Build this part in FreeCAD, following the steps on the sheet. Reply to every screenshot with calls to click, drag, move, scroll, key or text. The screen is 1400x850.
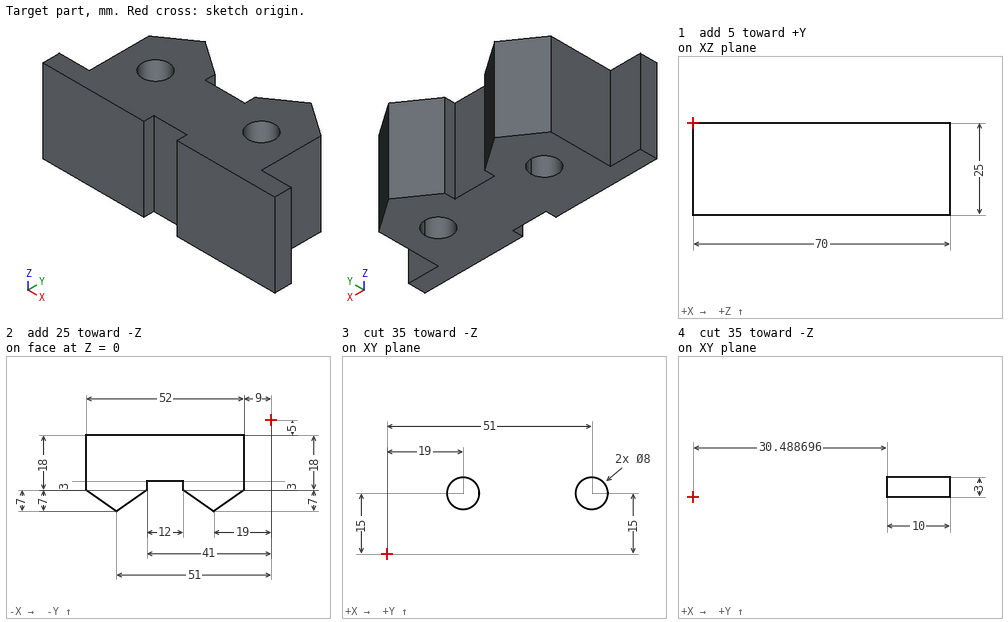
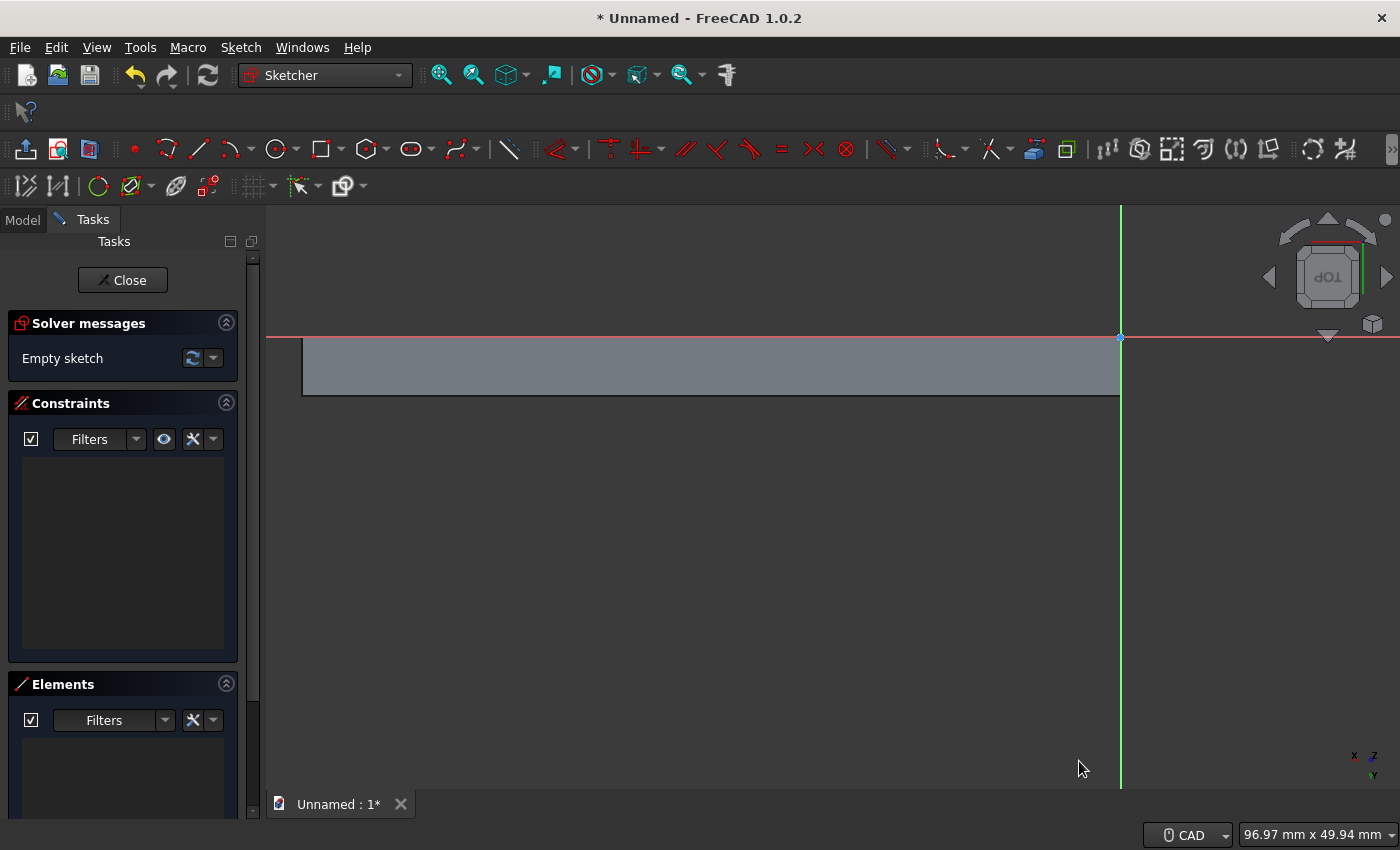
key(g)
key(m)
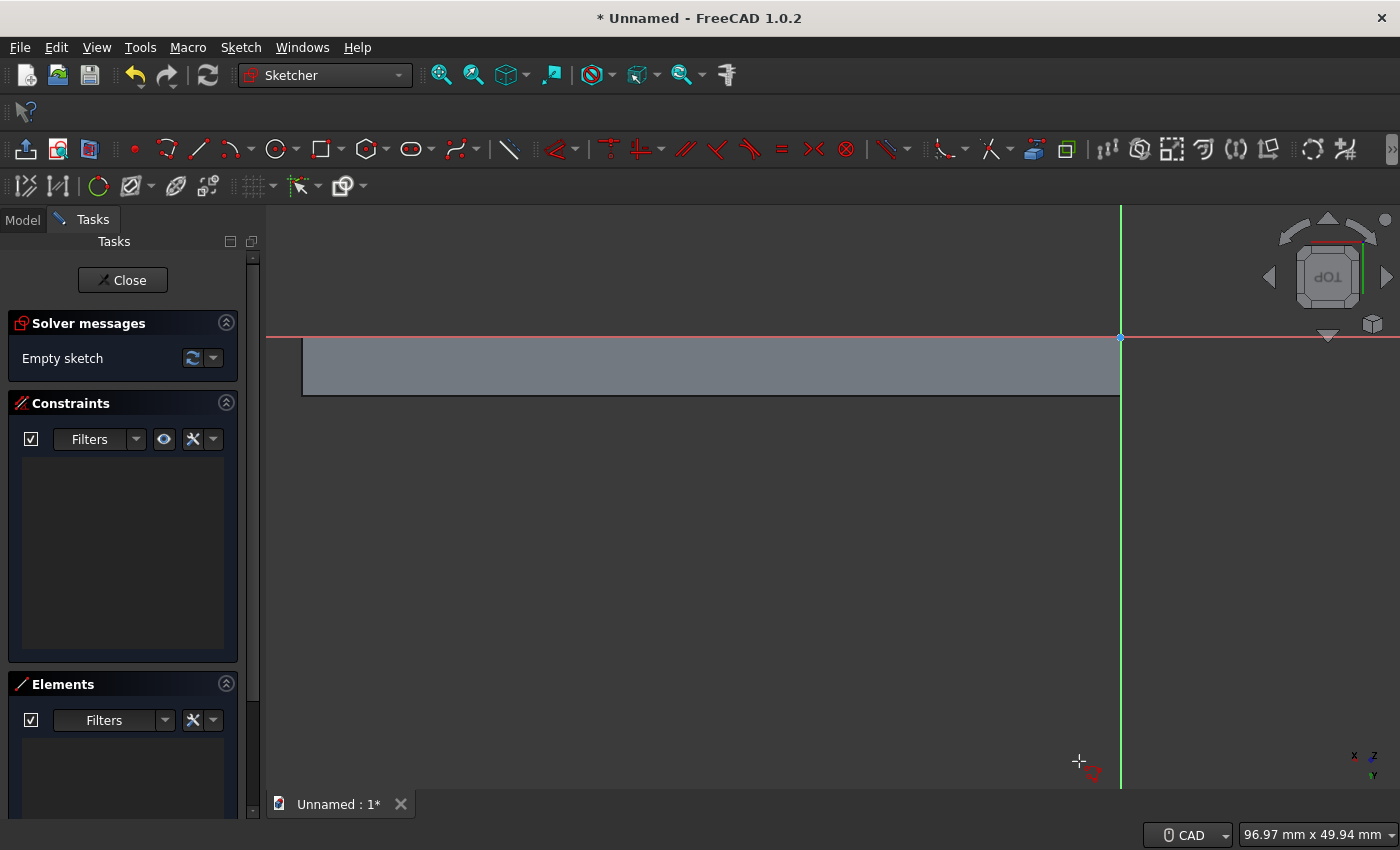
click(1016, 396)
click(408, 396)
click(408, 606)
click(525, 688)
click(641, 606)
click(641, 571)
click(782, 571)
click(782, 606)
click(899, 688)
click(1016, 606)
click(1016, 397)
key(Escape)
key(Escape)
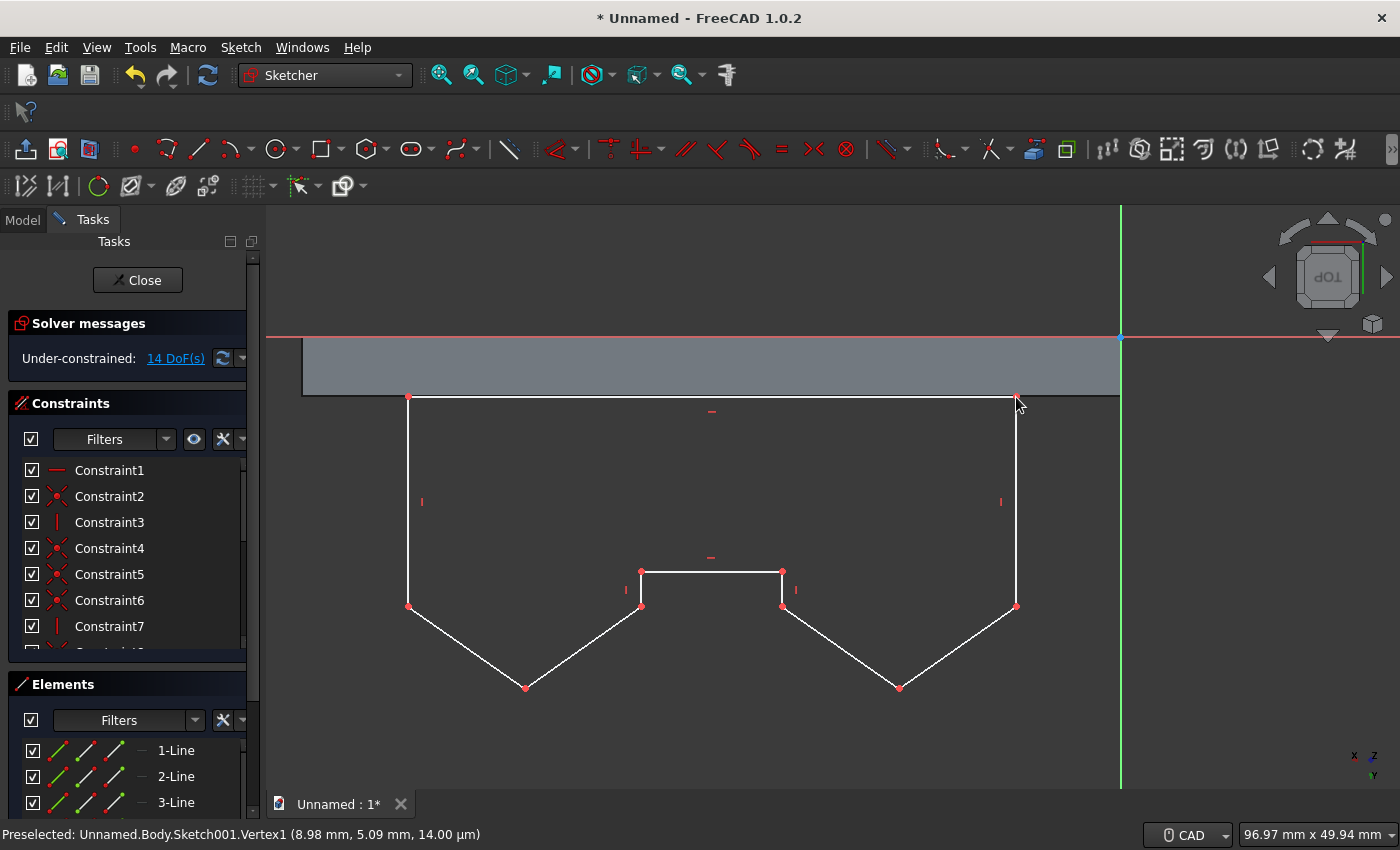
key(d)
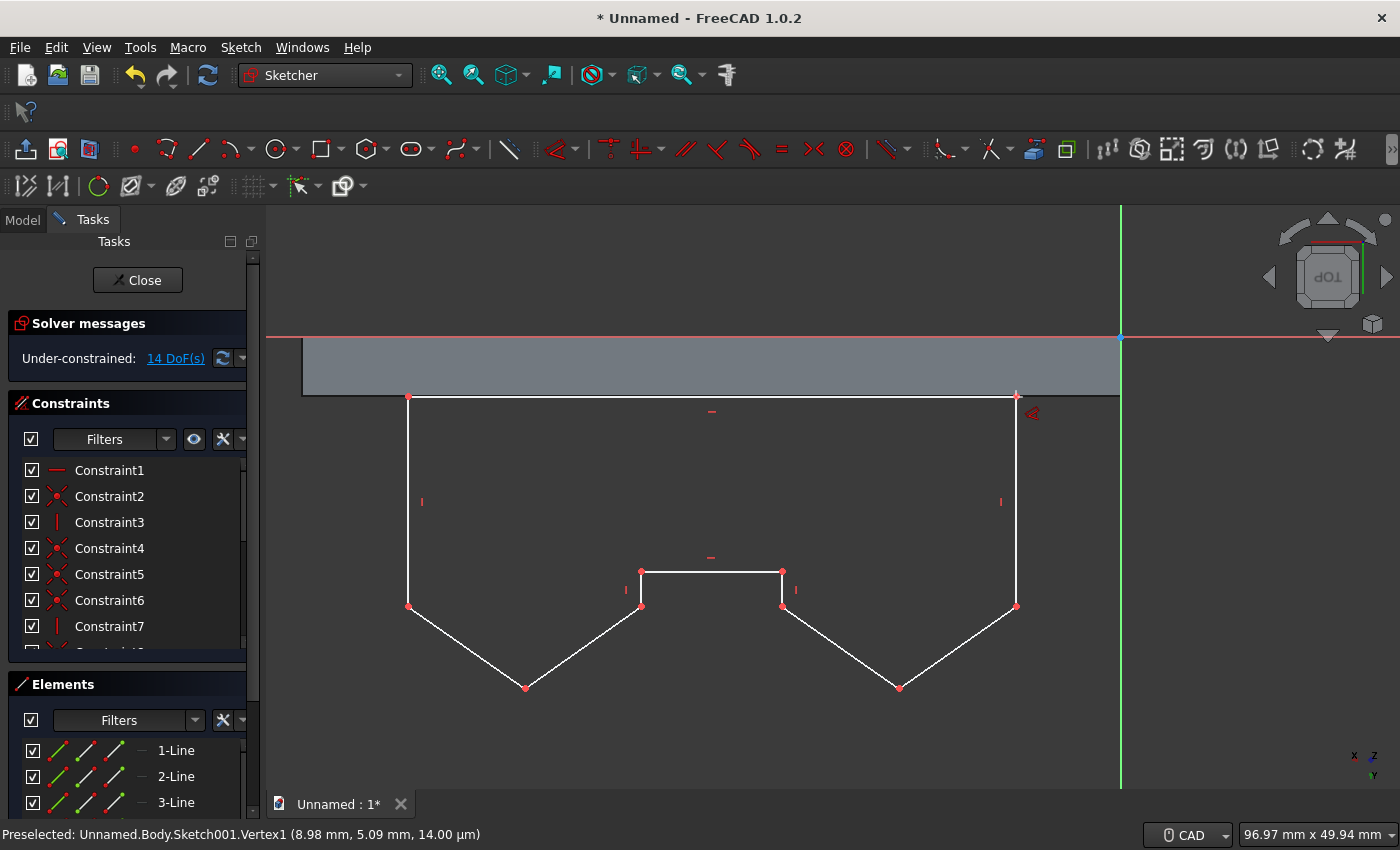
scroll(641, 597, up, 2)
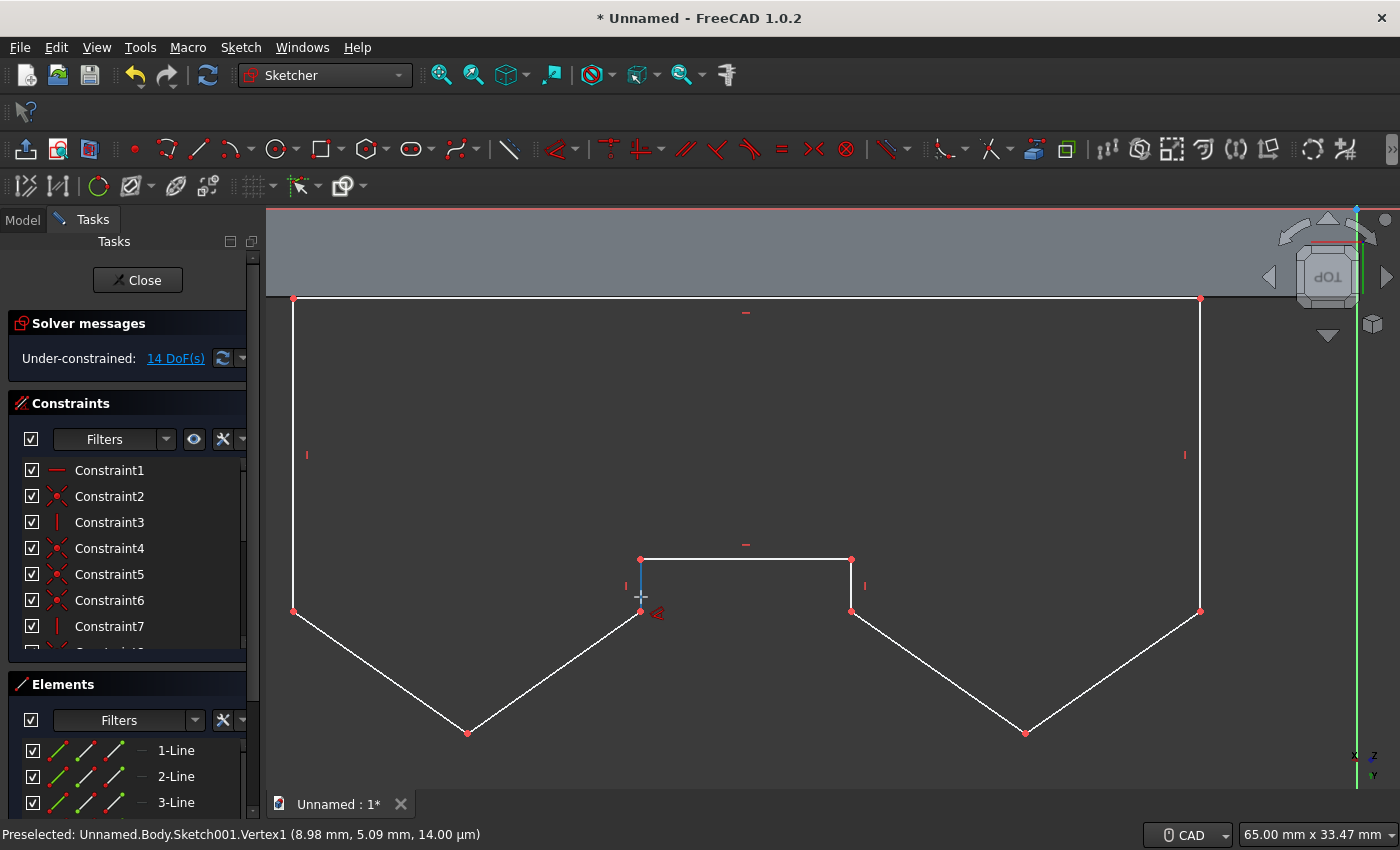
click(641, 596)
click(607, 585)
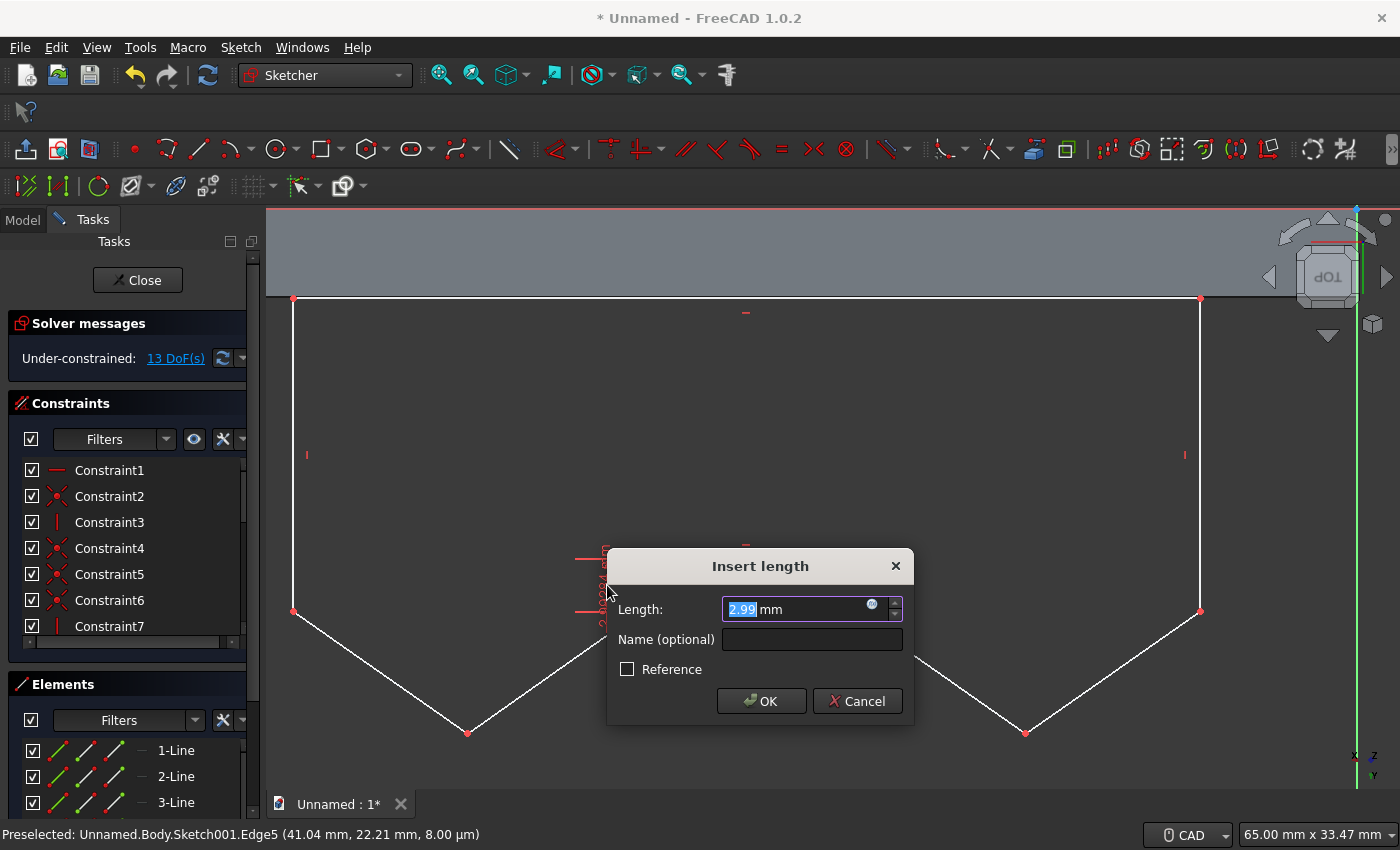
text(3)
key(Return)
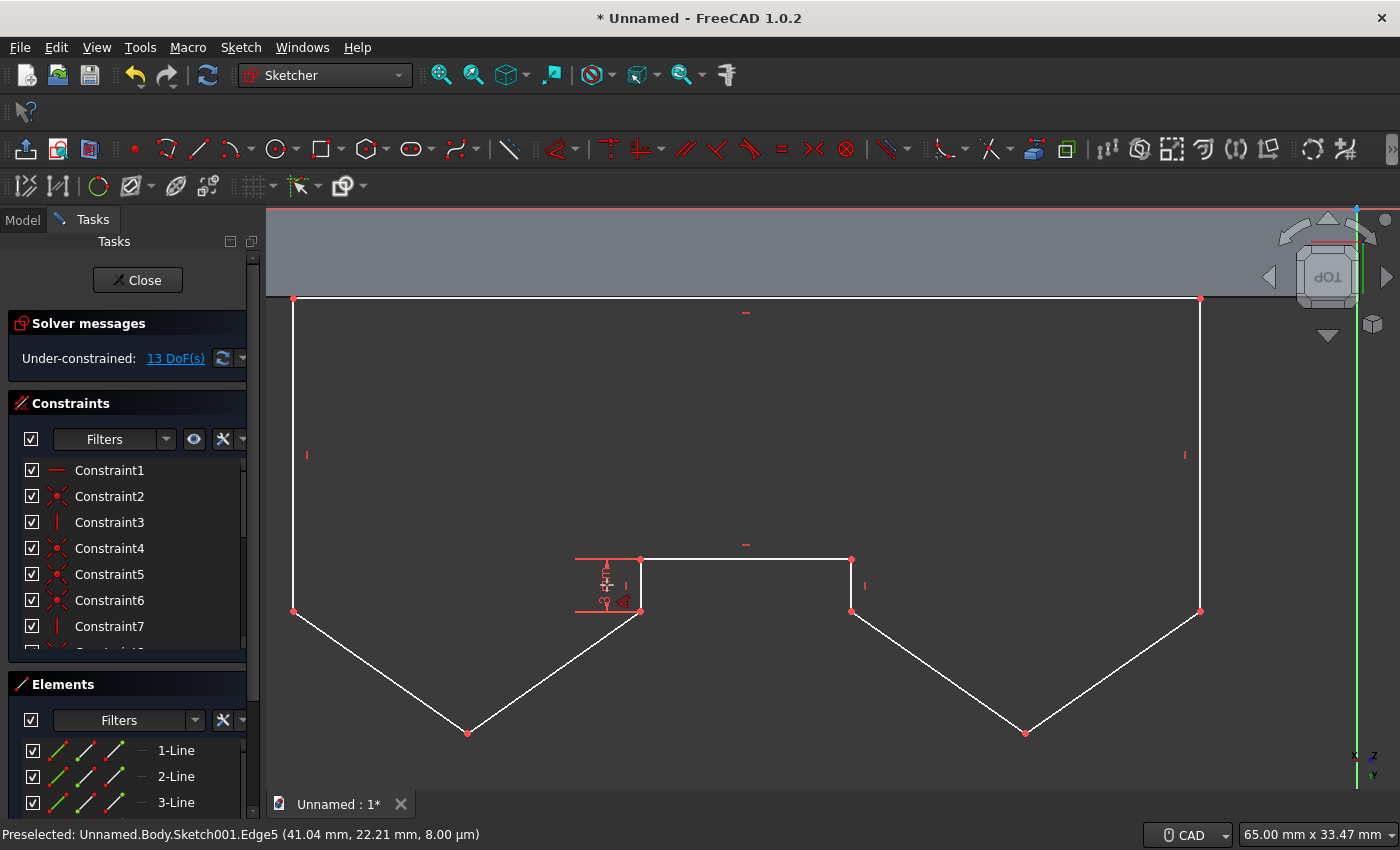
click(851, 575)
click(885, 585)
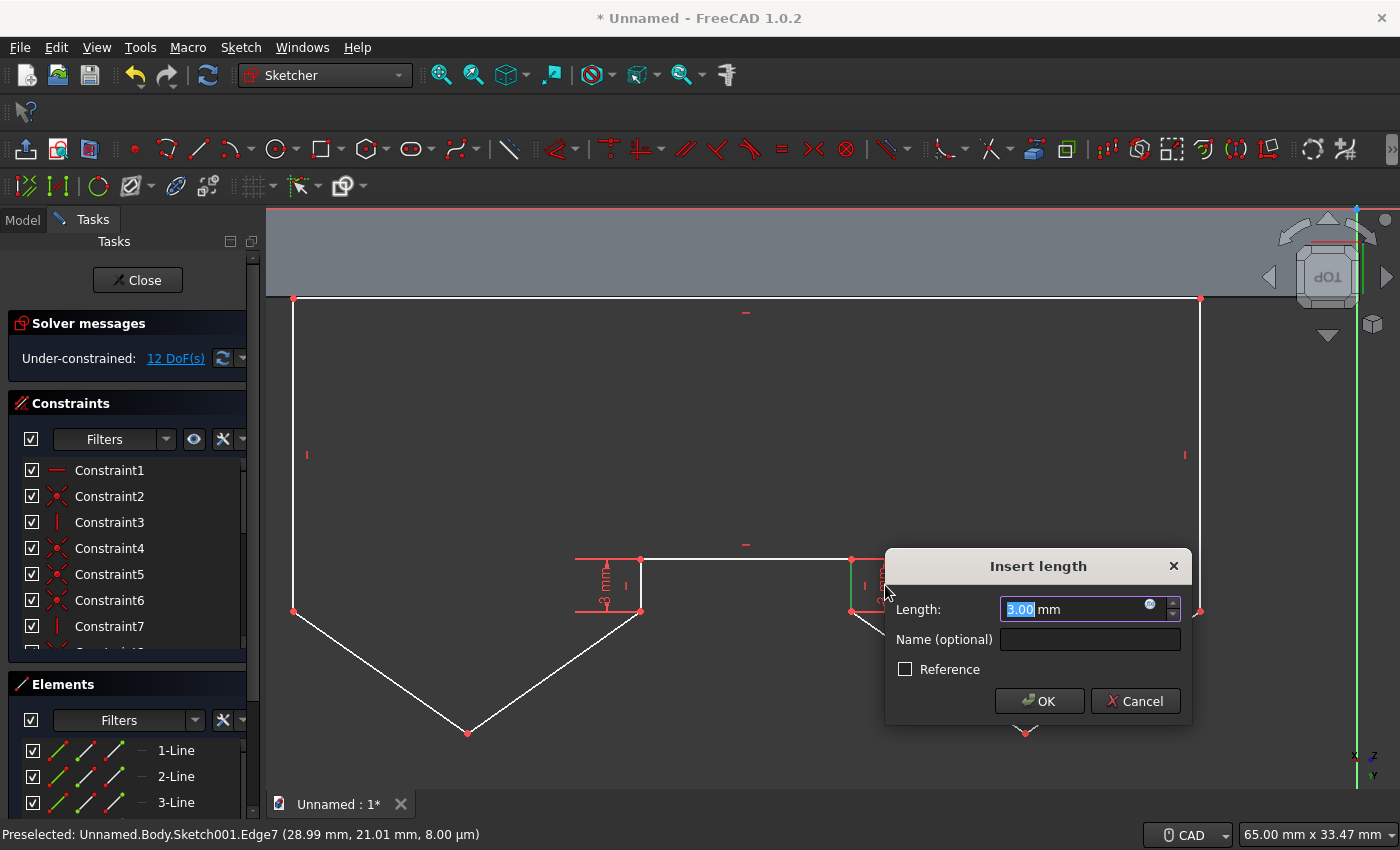
text(3)
key(Return)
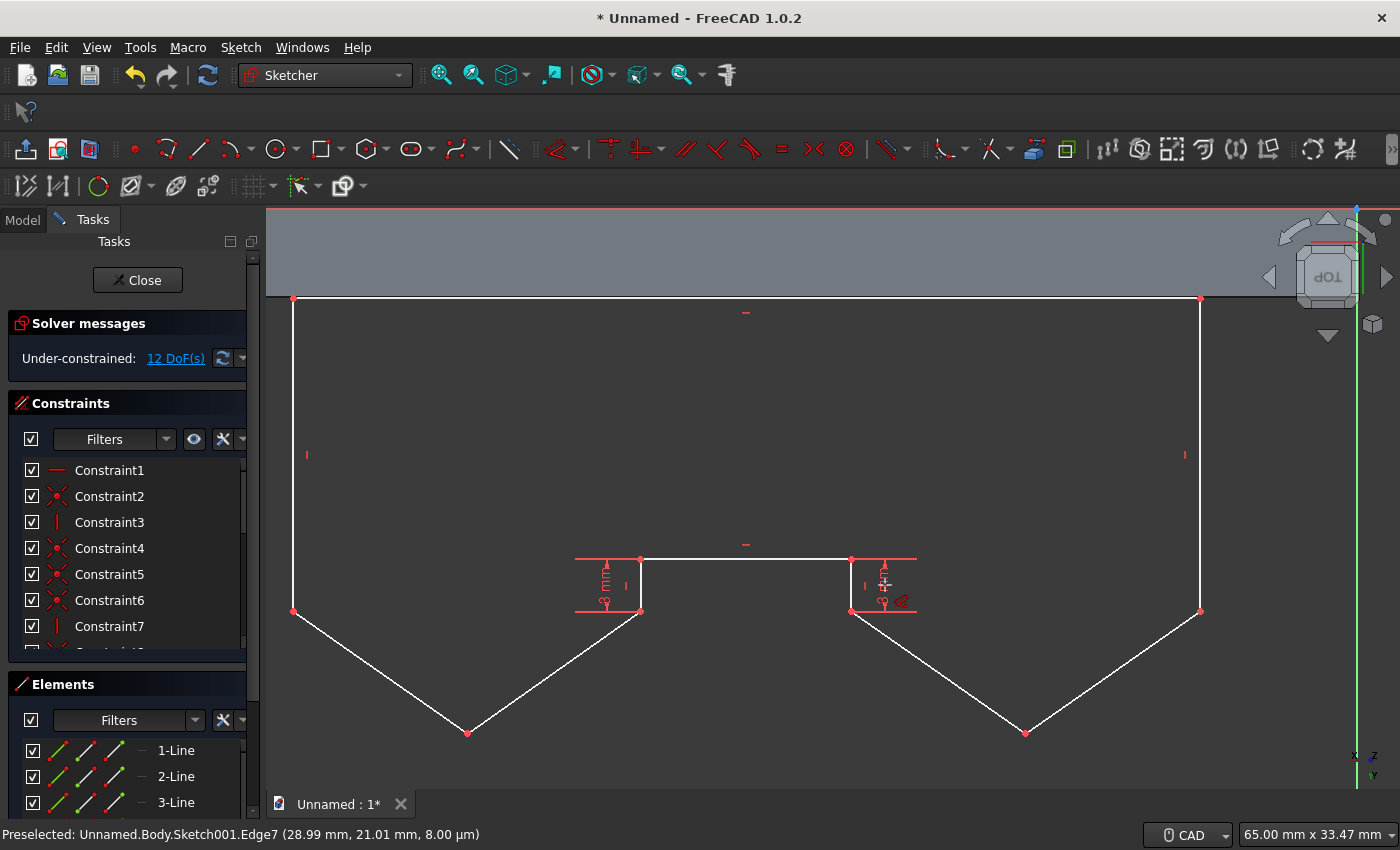
click(928, 298)
click(747, 264)